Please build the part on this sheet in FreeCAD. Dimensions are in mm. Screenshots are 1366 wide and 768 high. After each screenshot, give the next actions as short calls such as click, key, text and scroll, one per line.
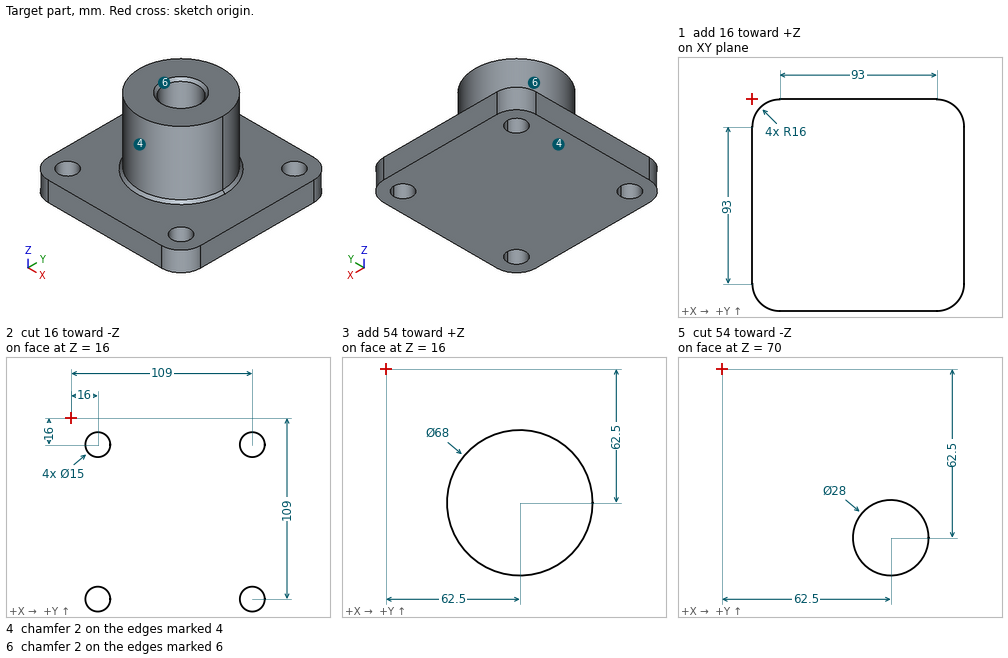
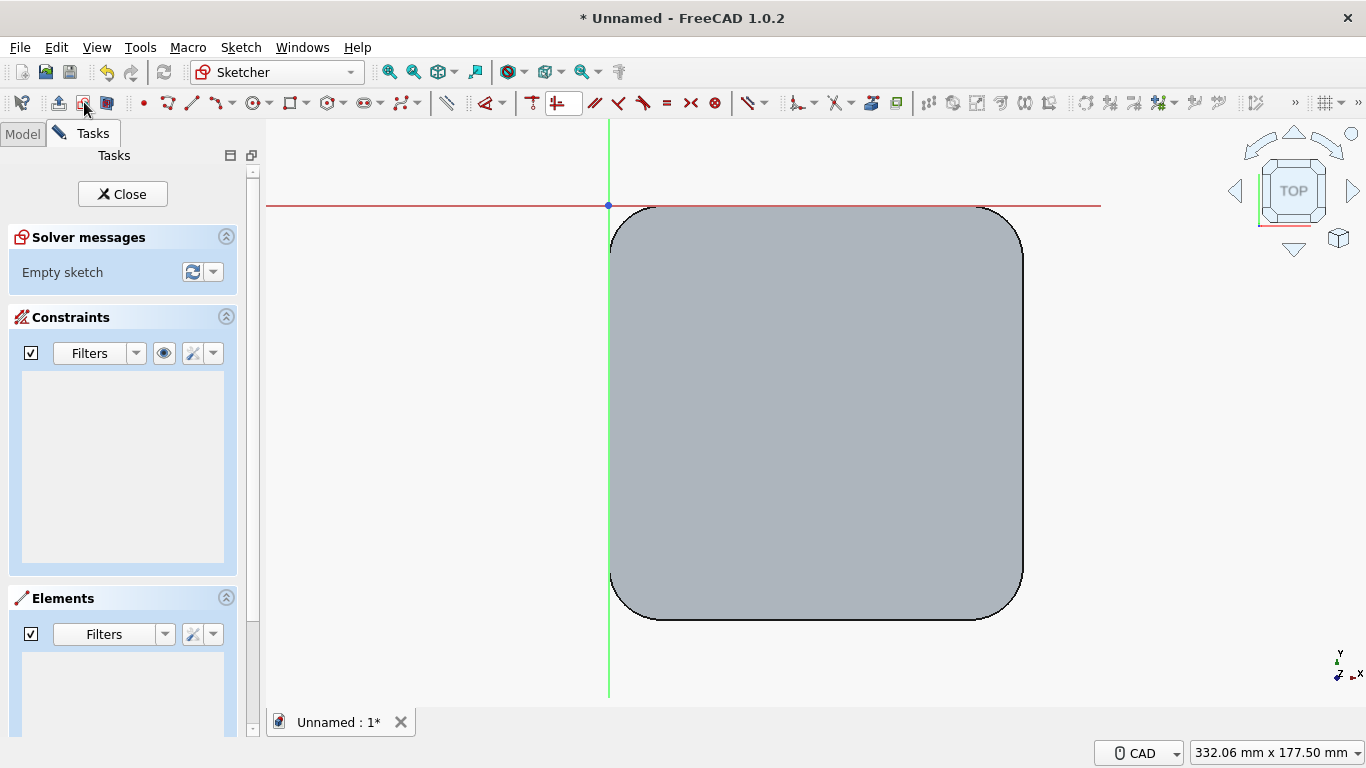
key(g)
key(c)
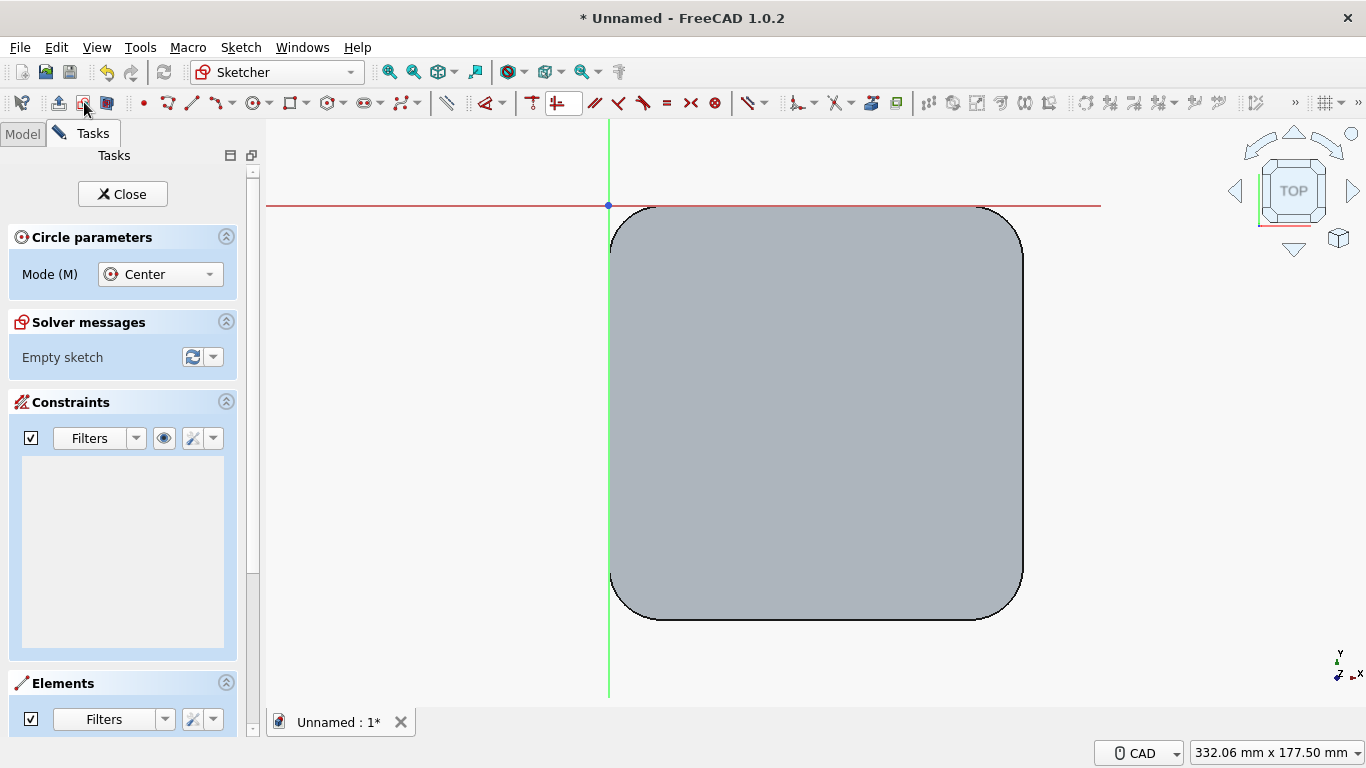
click(662, 259)
move(680, 241)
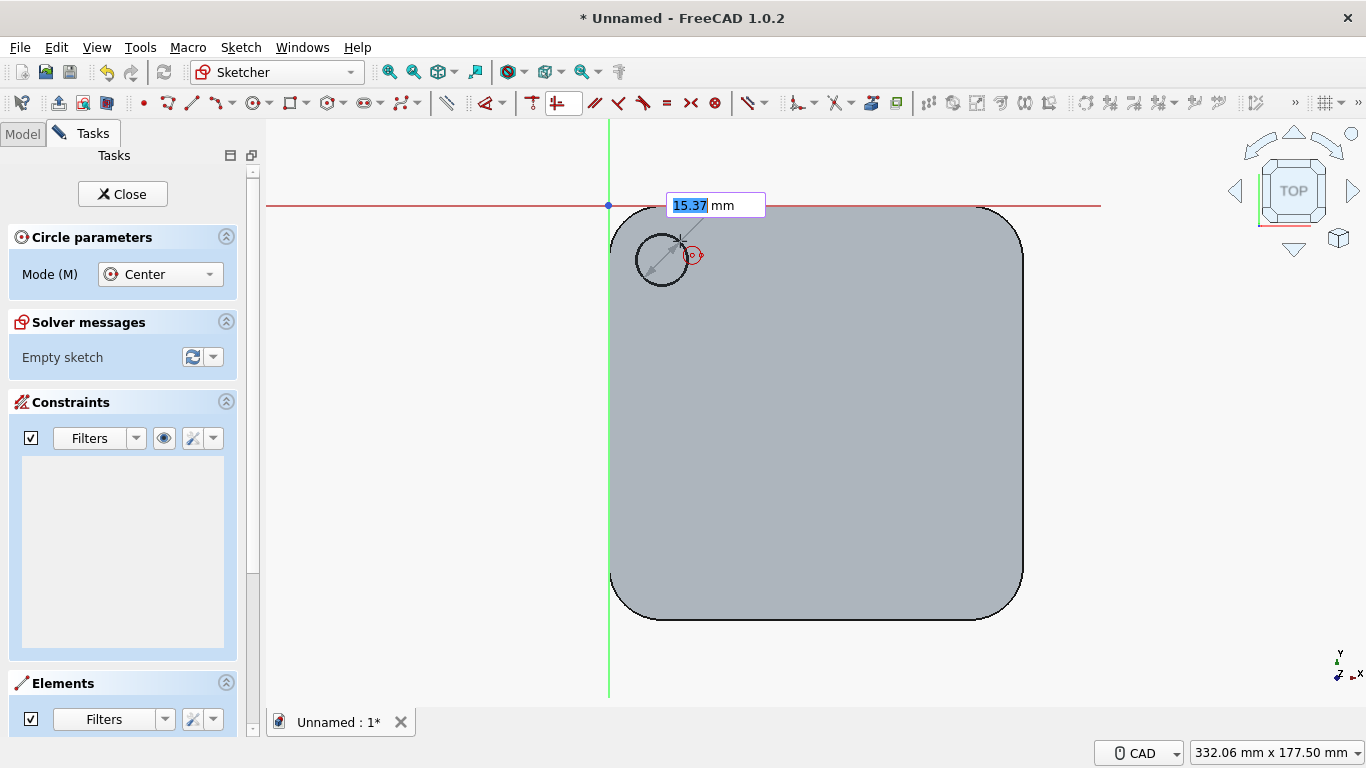
text(15)
key(Return)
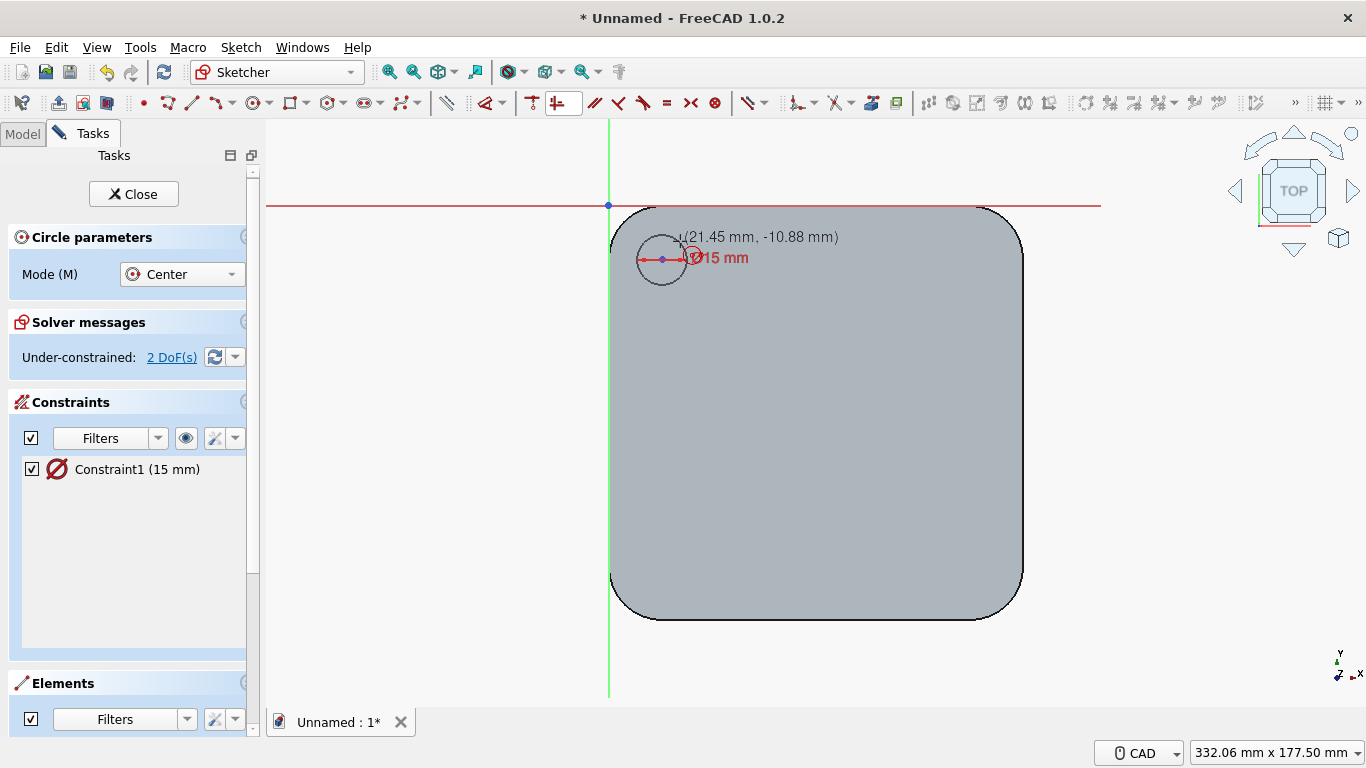
click(970, 259)
move(988, 241)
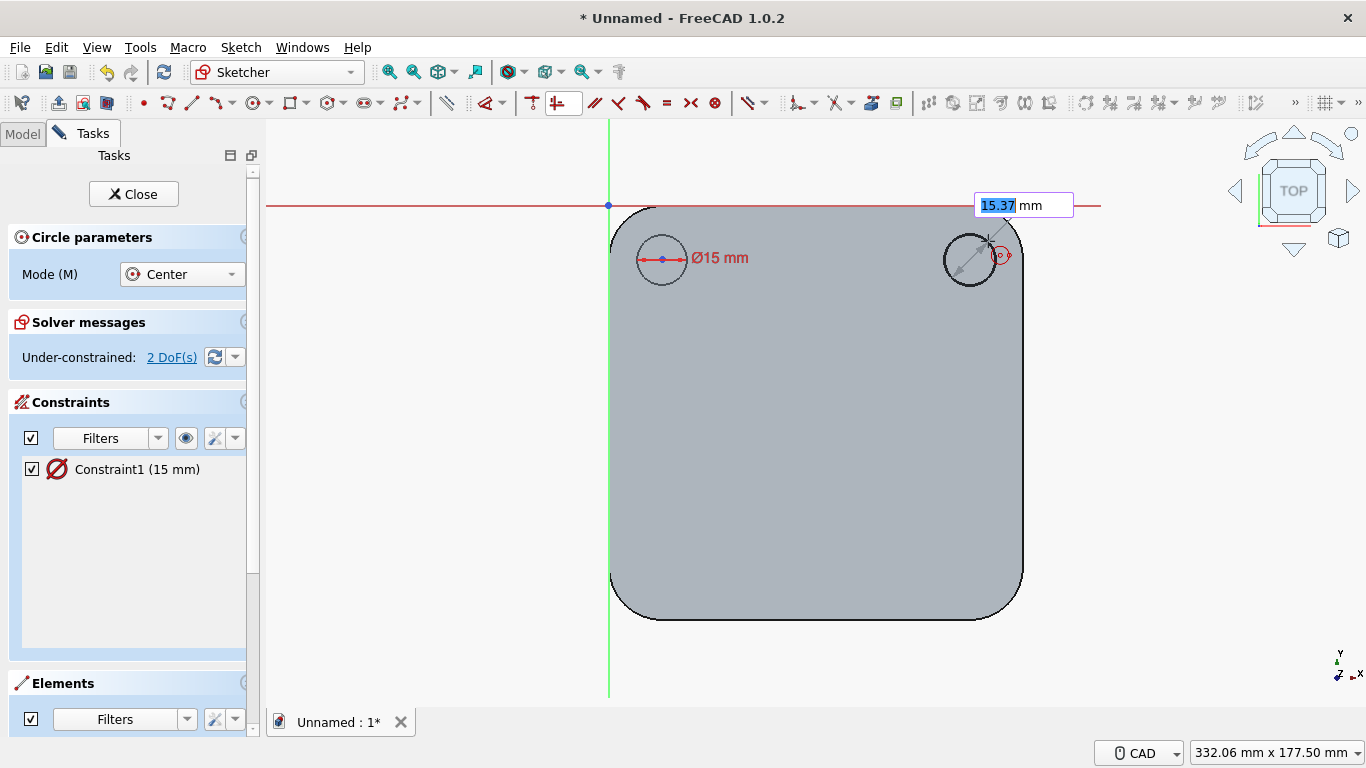
text(15)
key(Return)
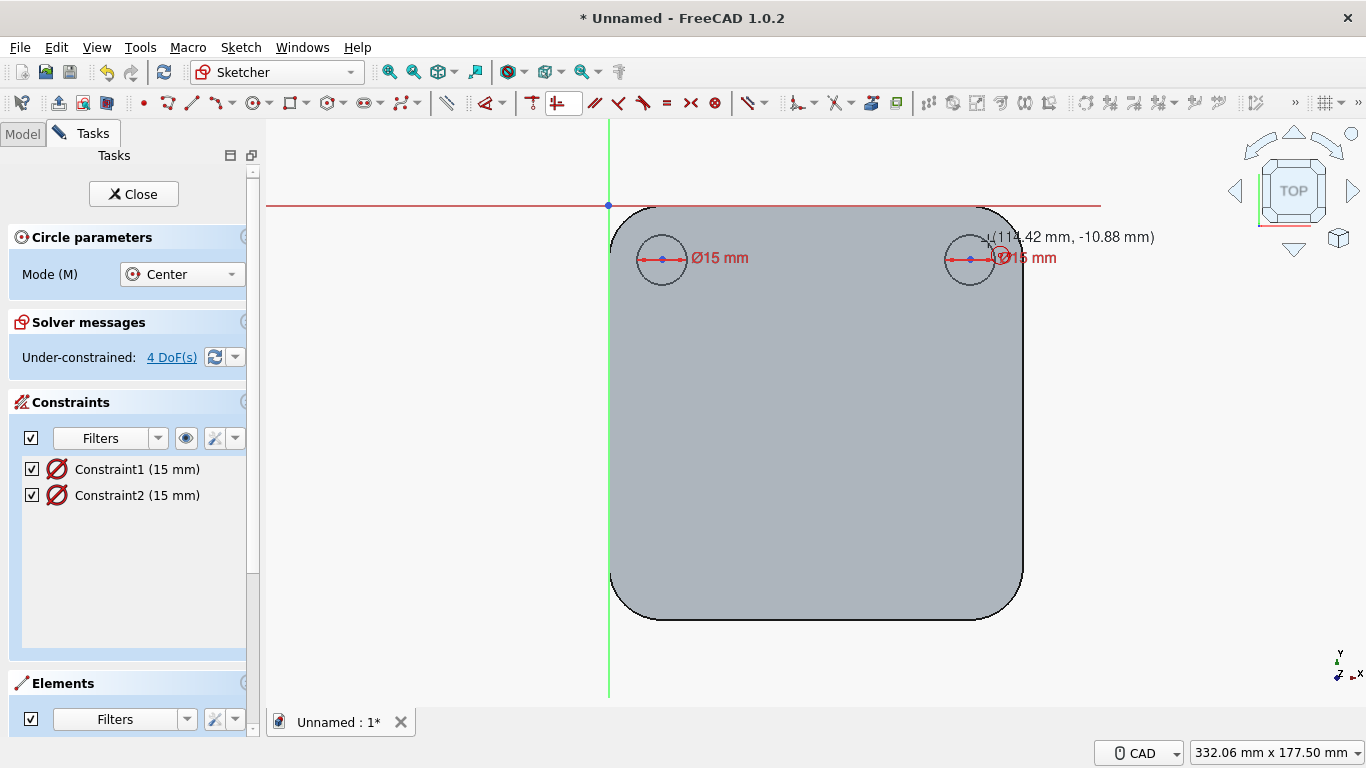
click(970, 567)
move(988, 549)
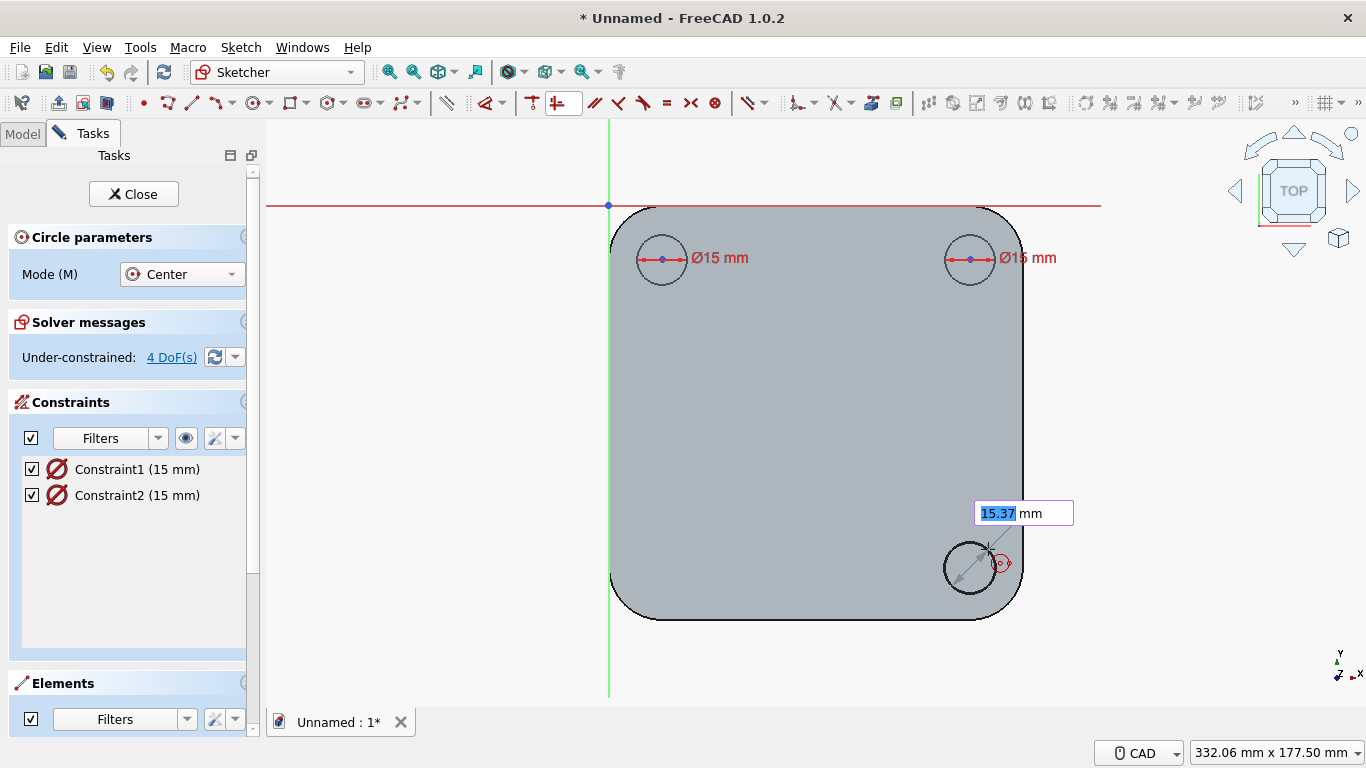
text(15)
key(Return)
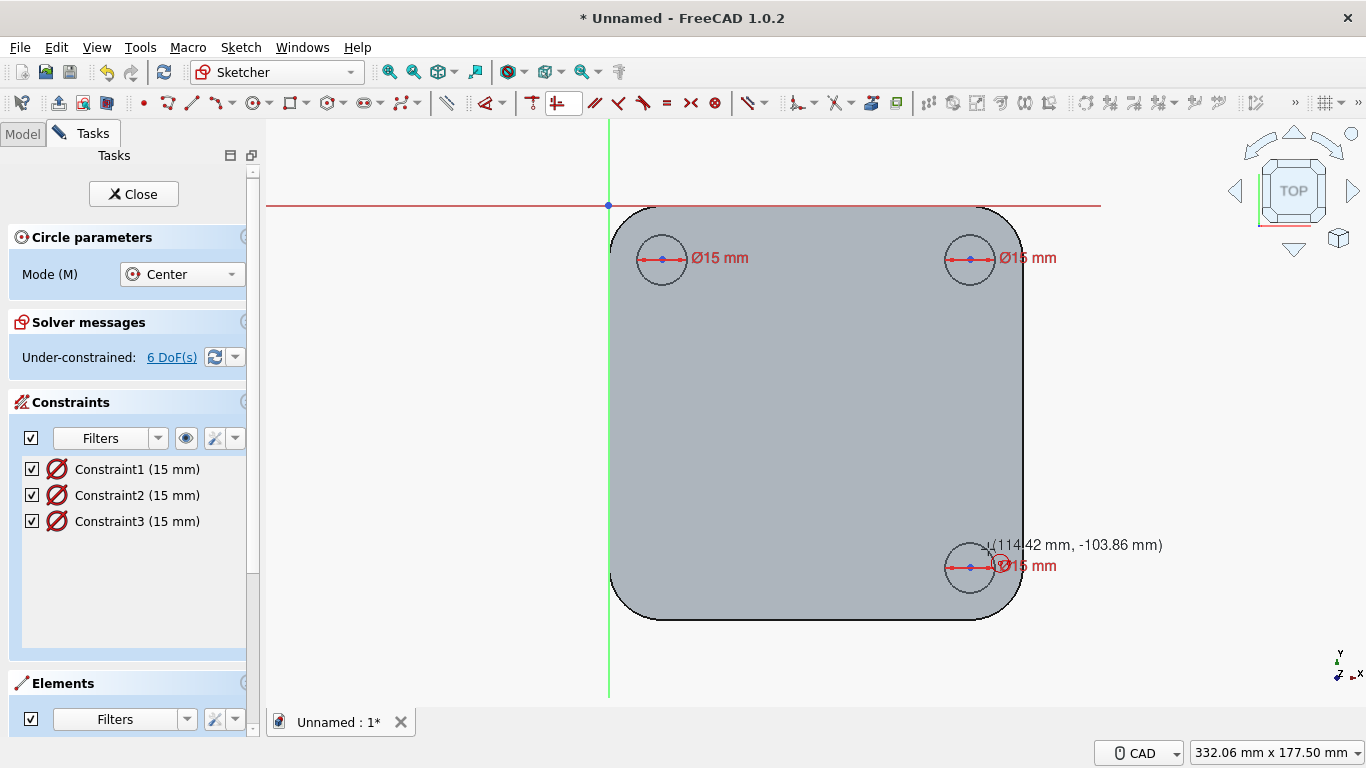
click(662, 567)
move(680, 549)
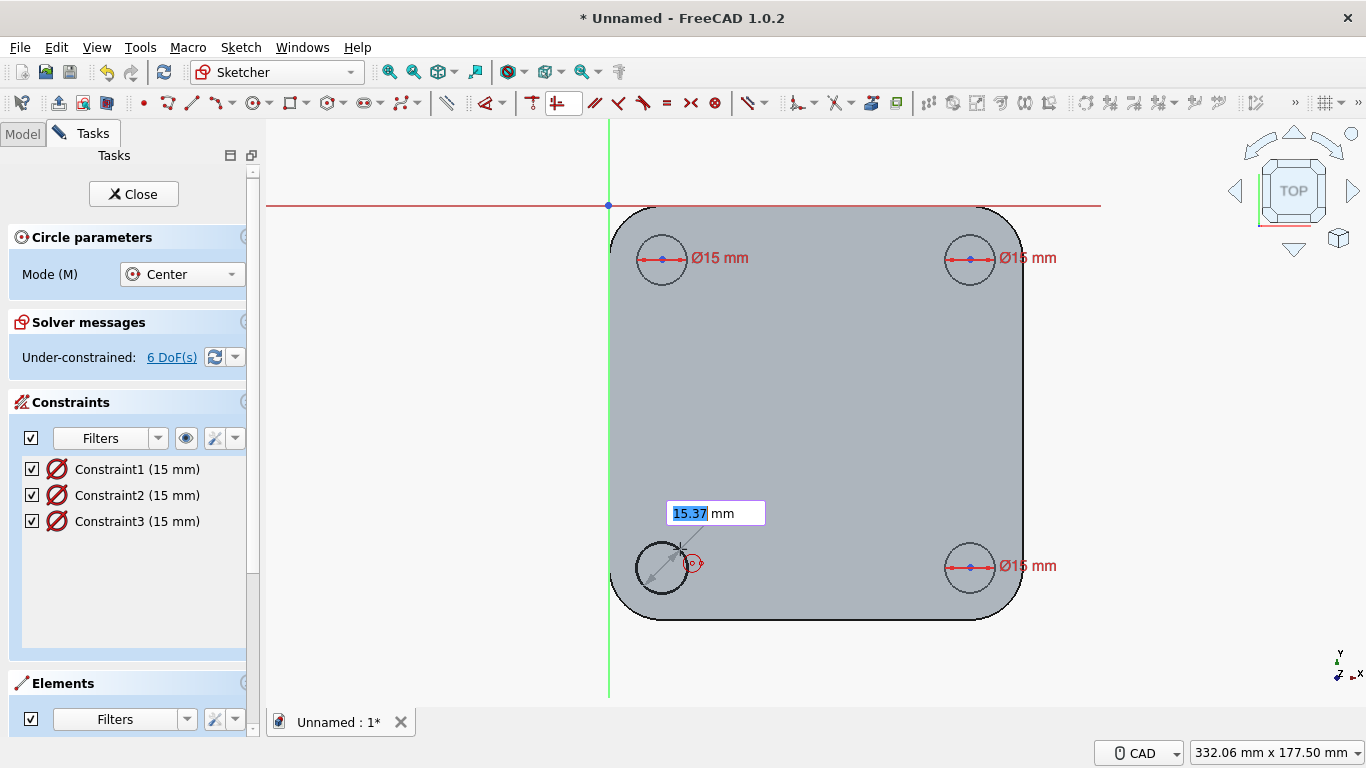
text(15)
key(Return)
key(Escape)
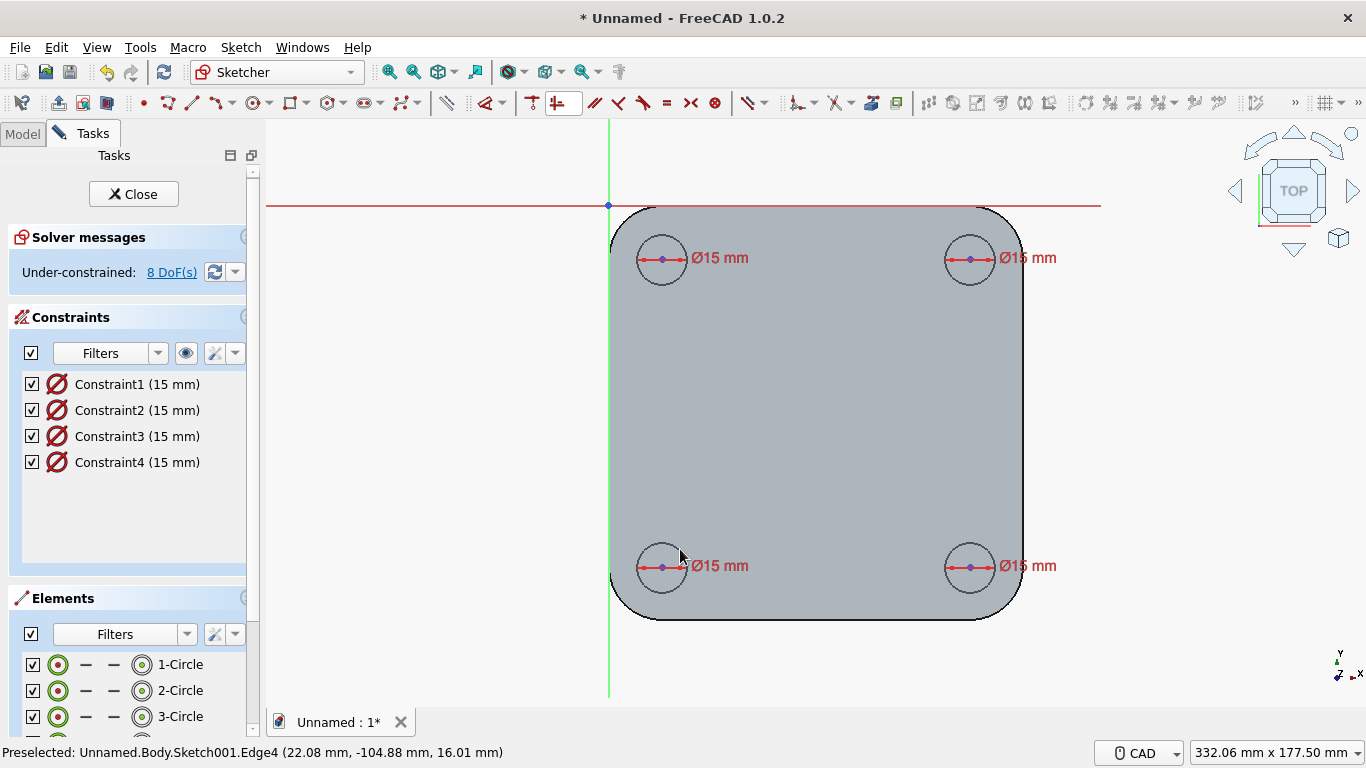
click(662, 260)